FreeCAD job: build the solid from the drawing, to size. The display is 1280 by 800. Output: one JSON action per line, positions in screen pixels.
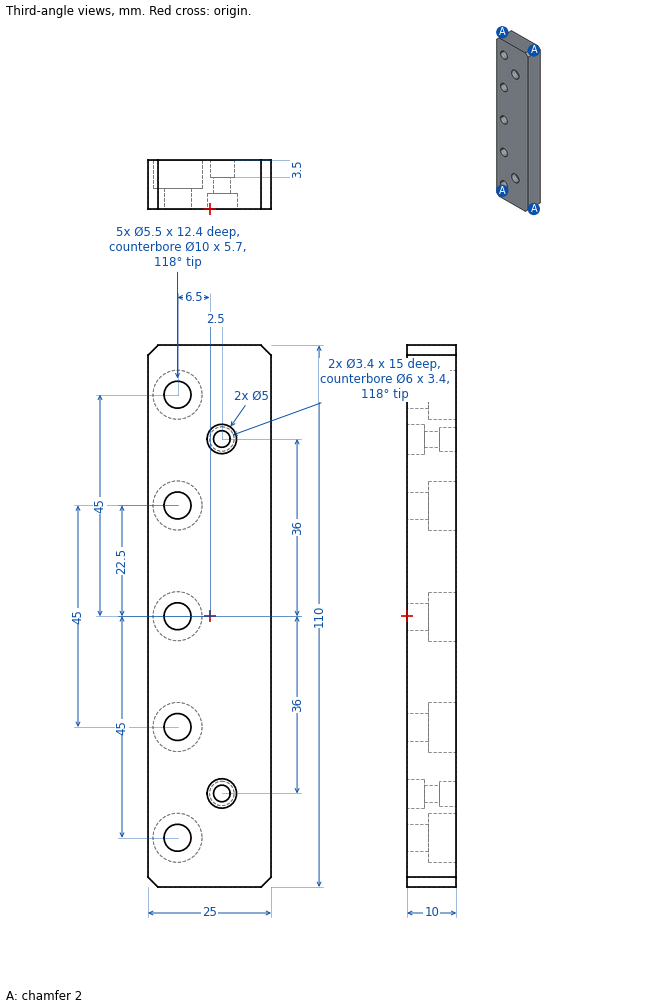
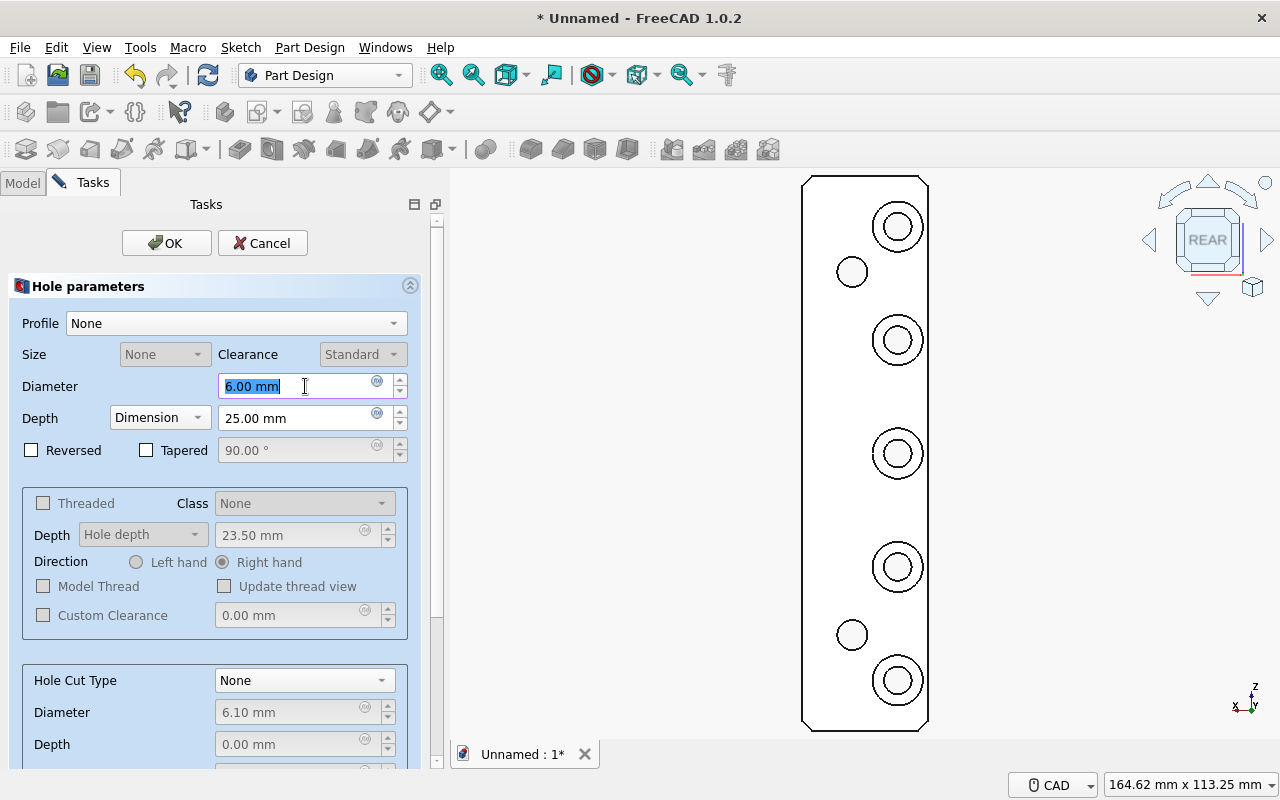
{"action": "type", "text": "3.4"}
{"action": "key", "text": "Tab"}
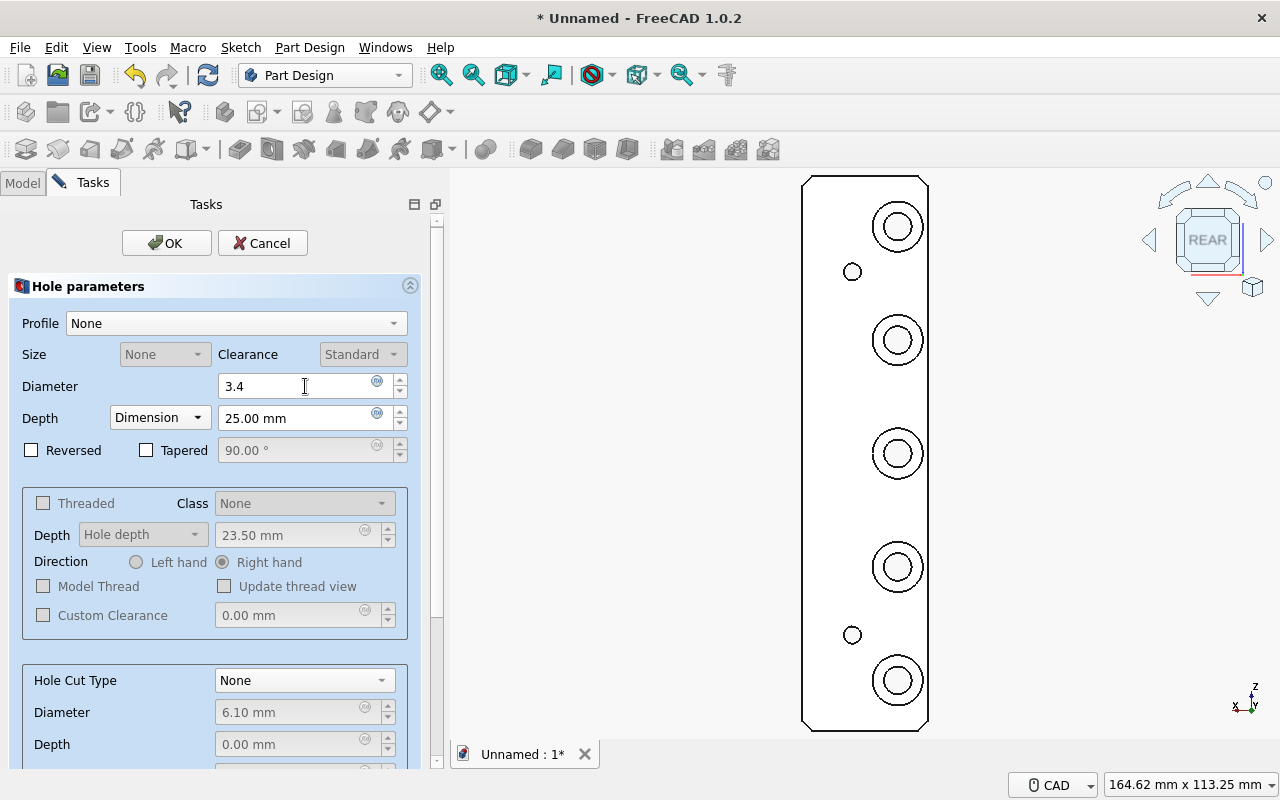
{"action": "triple_click", "coordinate": [305, 418]}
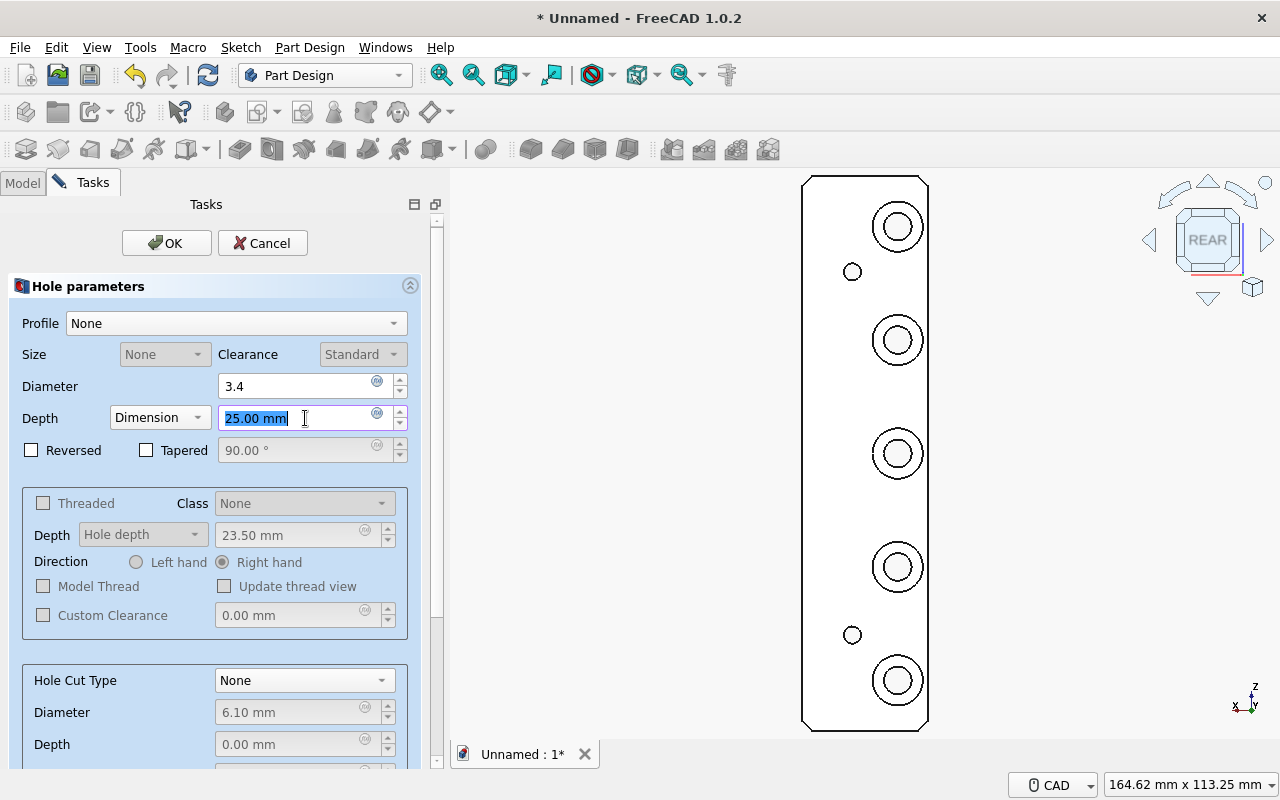
{"action": "type", "text": "15"}
{"action": "key", "text": "Tab"}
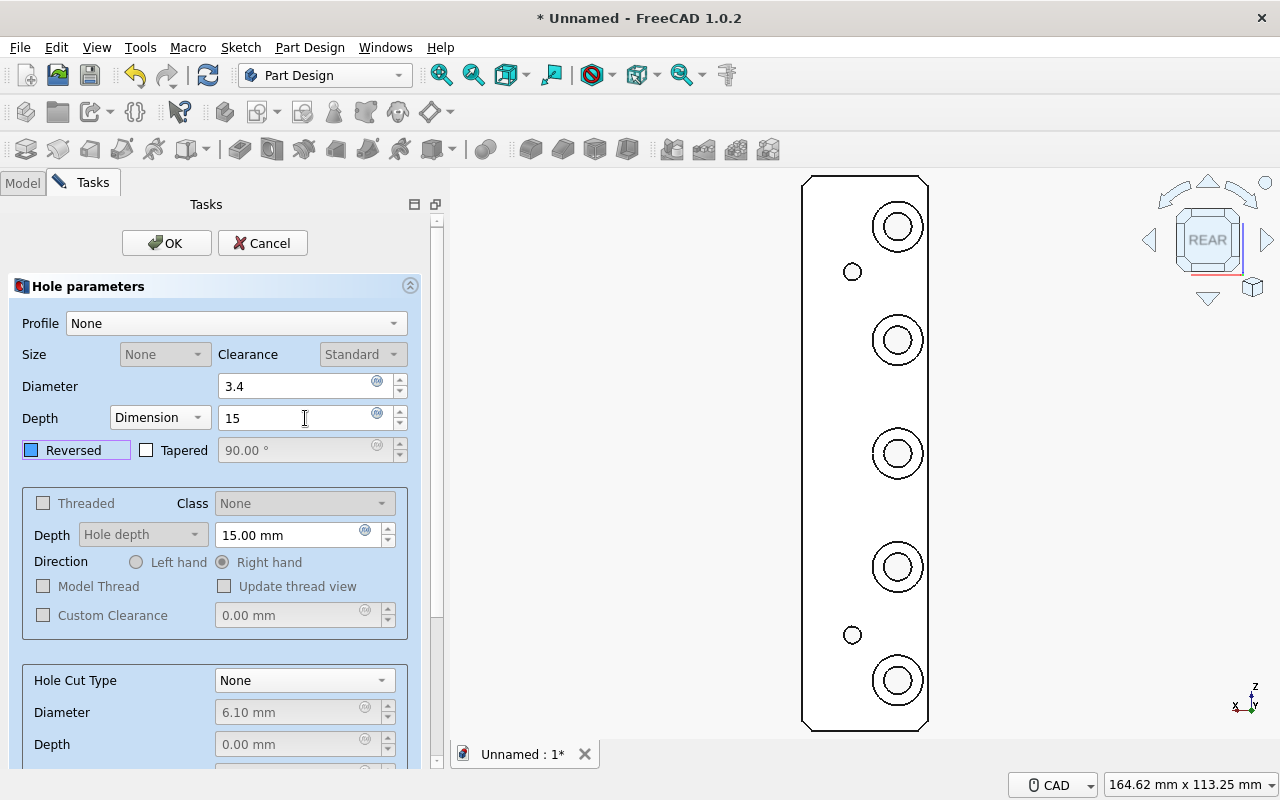
{"action": "left_click", "coordinate": [306, 680]}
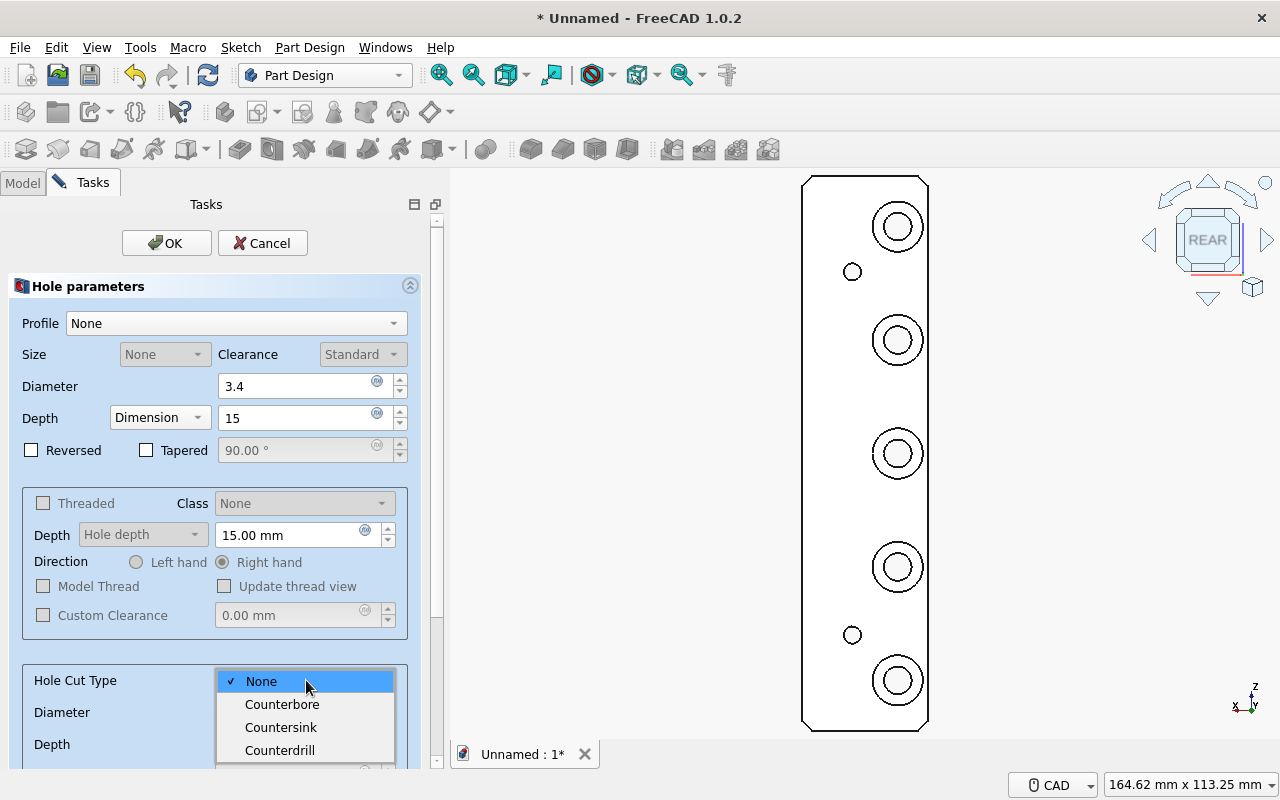
{"action": "left_click", "coordinate": [304, 704]}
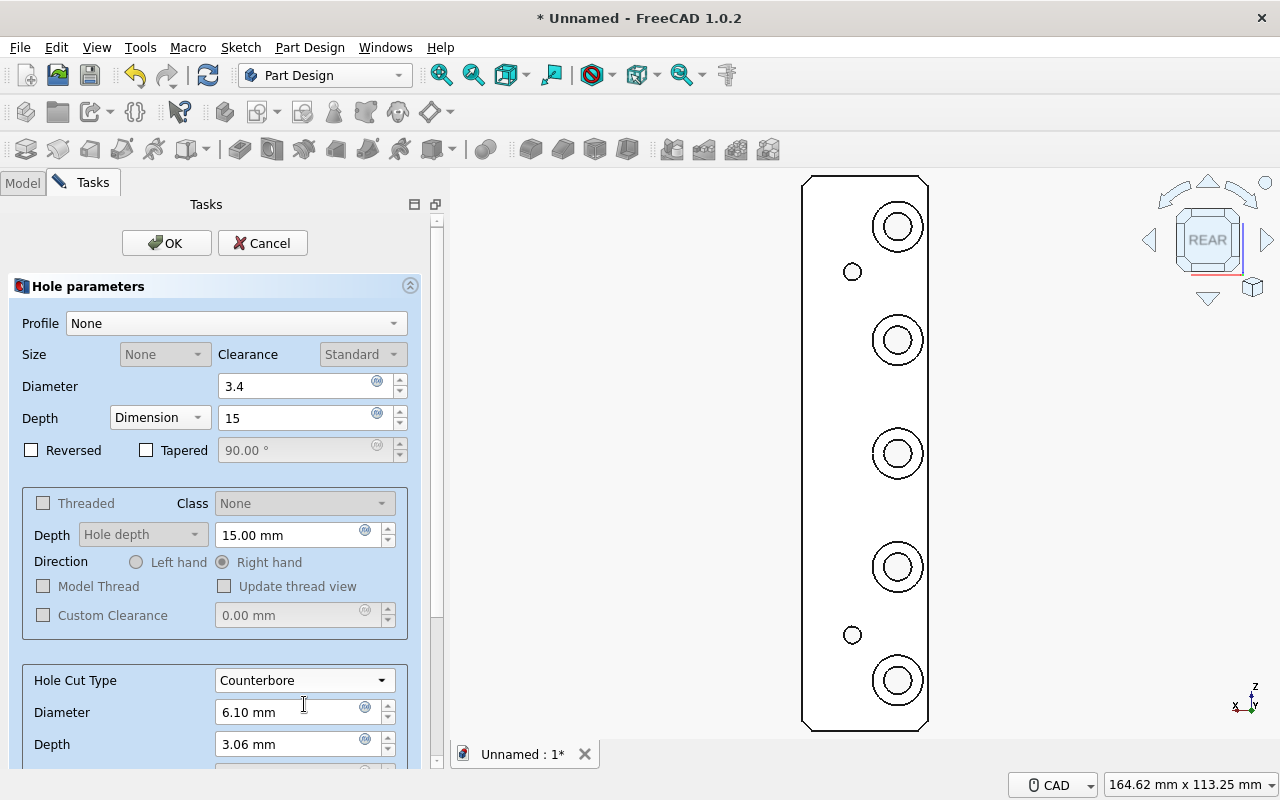
{"action": "triple_click", "coordinate": [298, 712]}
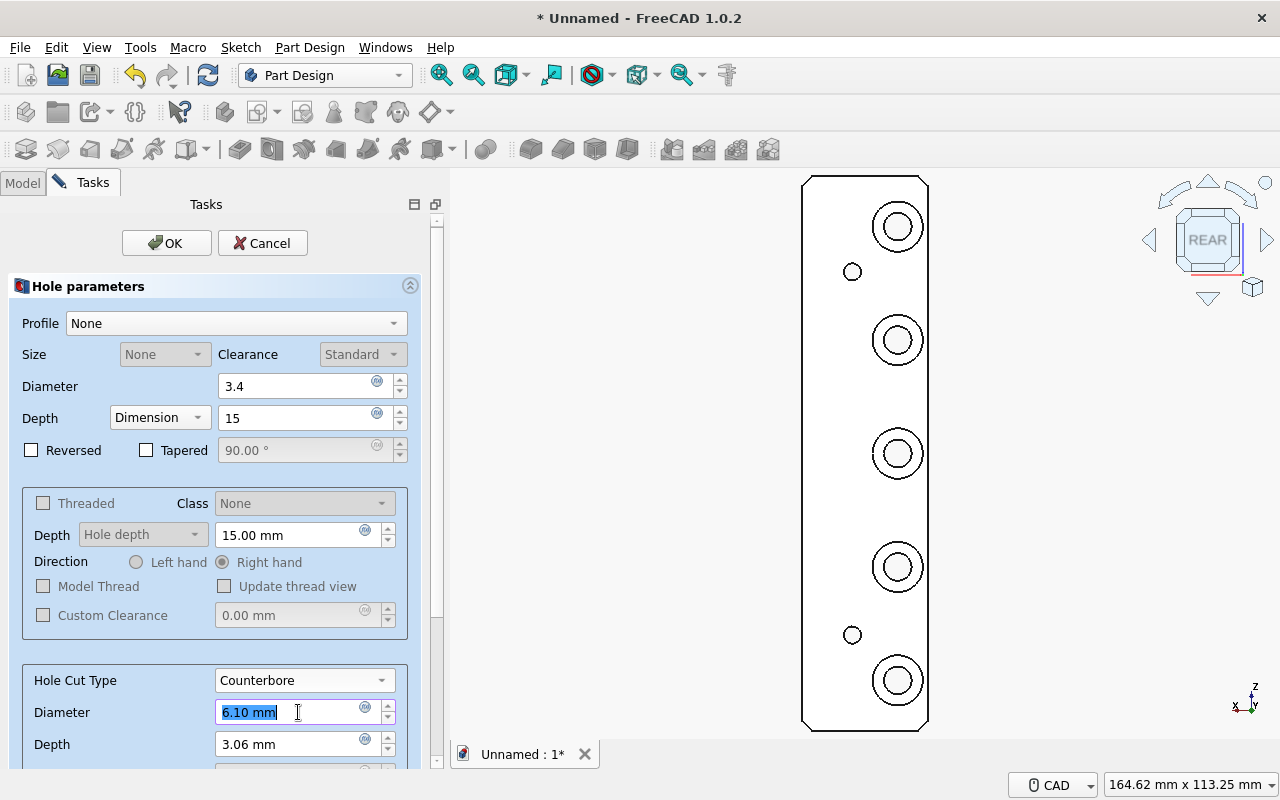
{"action": "type", "text": "6"}
{"action": "key", "text": "Tab"}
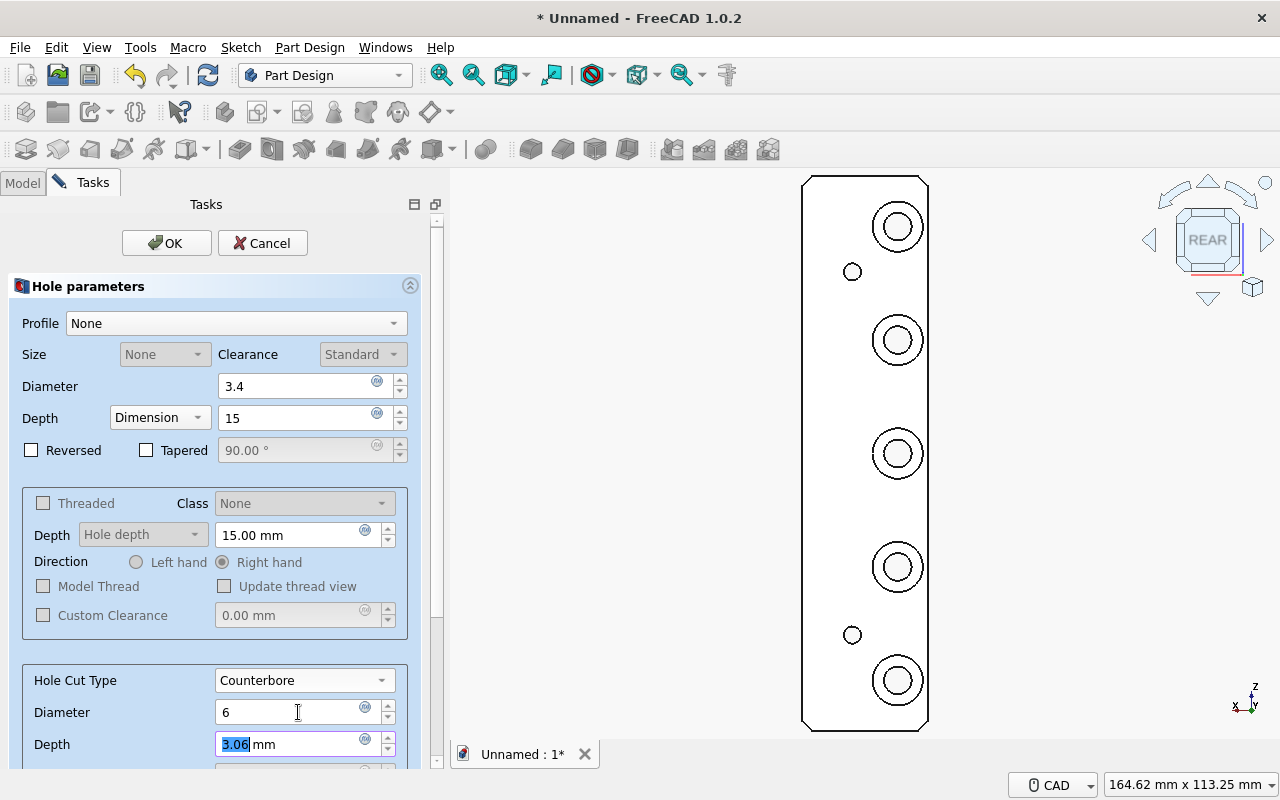
{"action": "type", "text": "3.4"}
{"action": "key", "text": "Tab"}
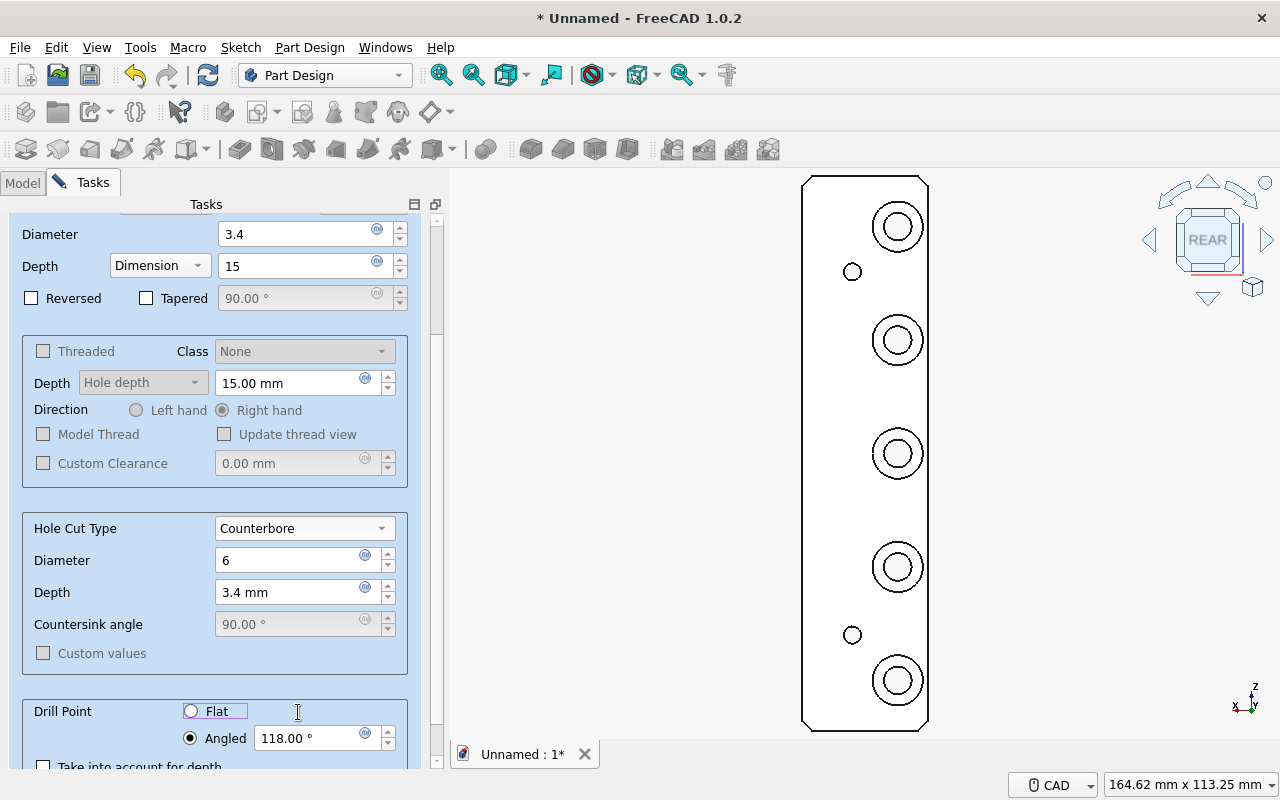
{"action": "scroll", "coordinate": [437, 491], "scroll_direction": "up", "scroll_amount": 4}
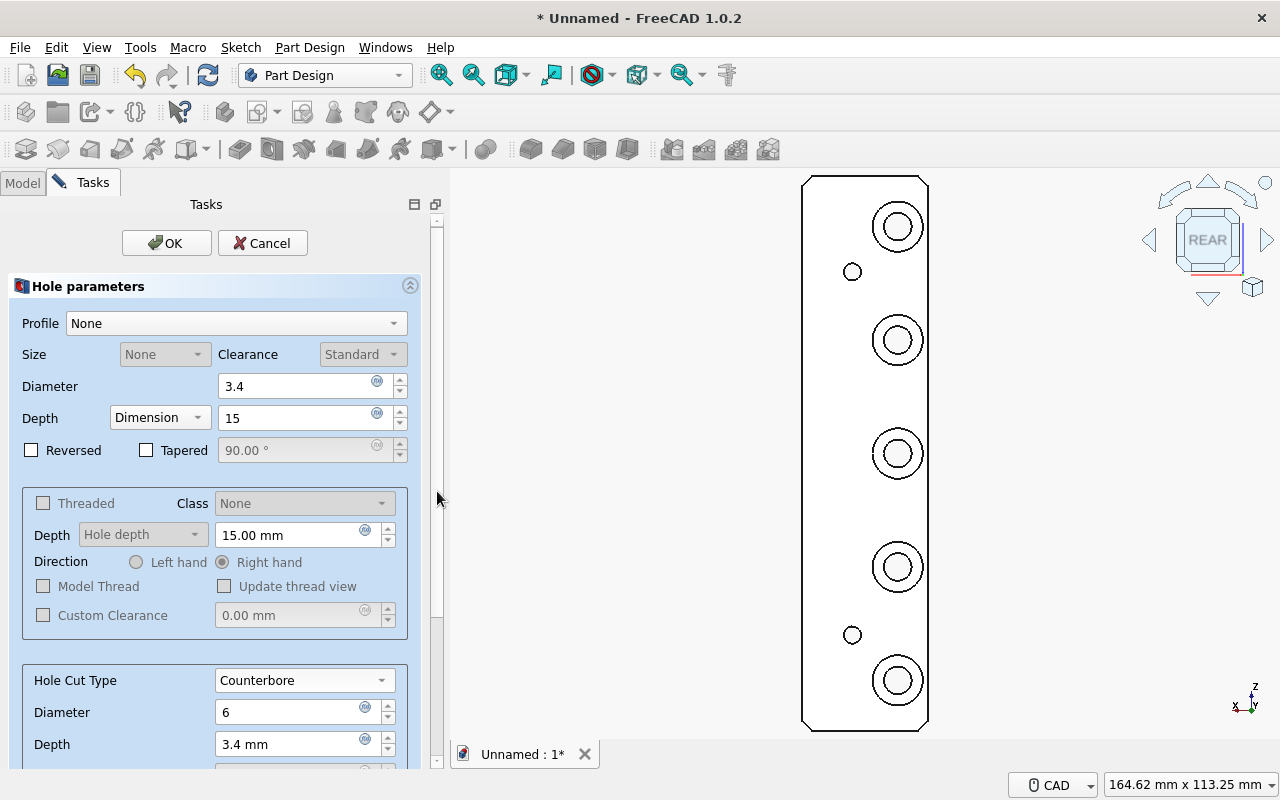
{"action": "left_click", "coordinate": [167, 243]}